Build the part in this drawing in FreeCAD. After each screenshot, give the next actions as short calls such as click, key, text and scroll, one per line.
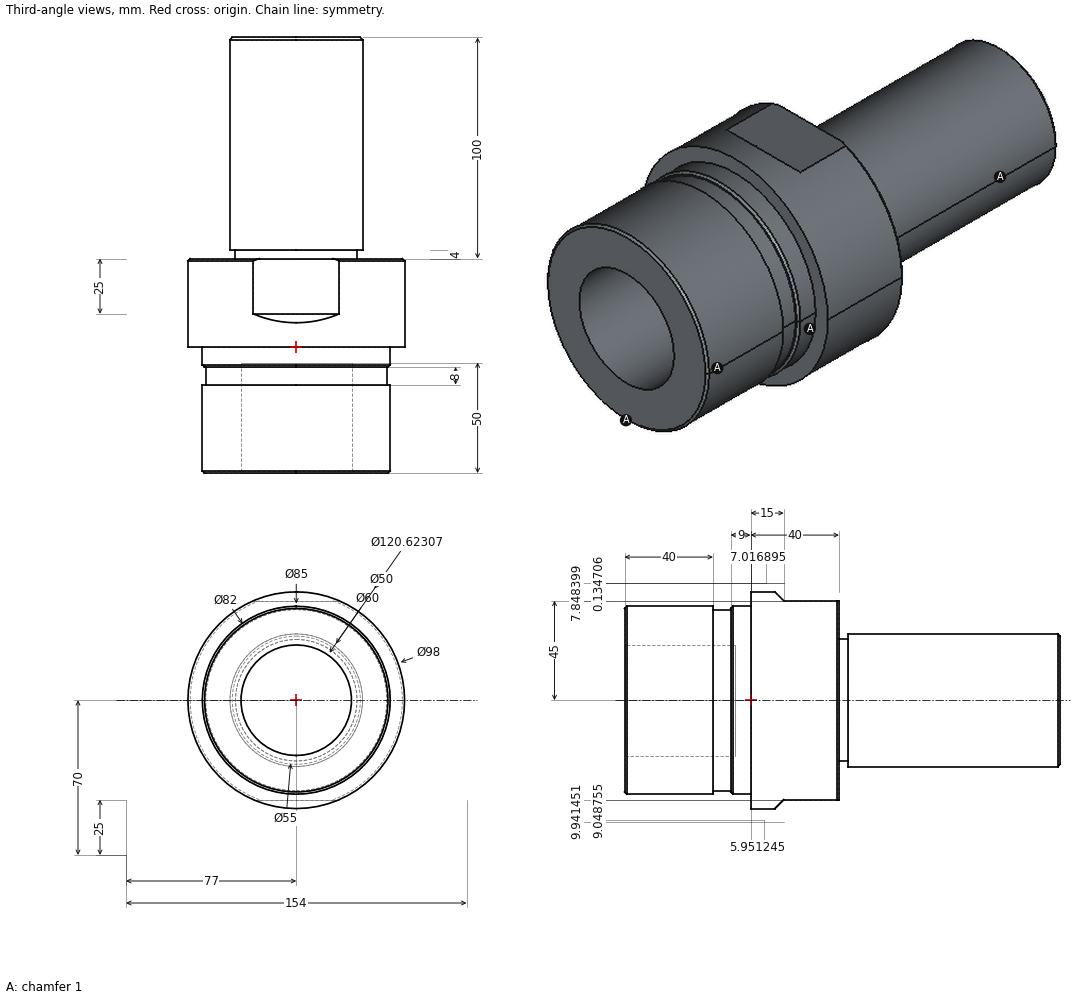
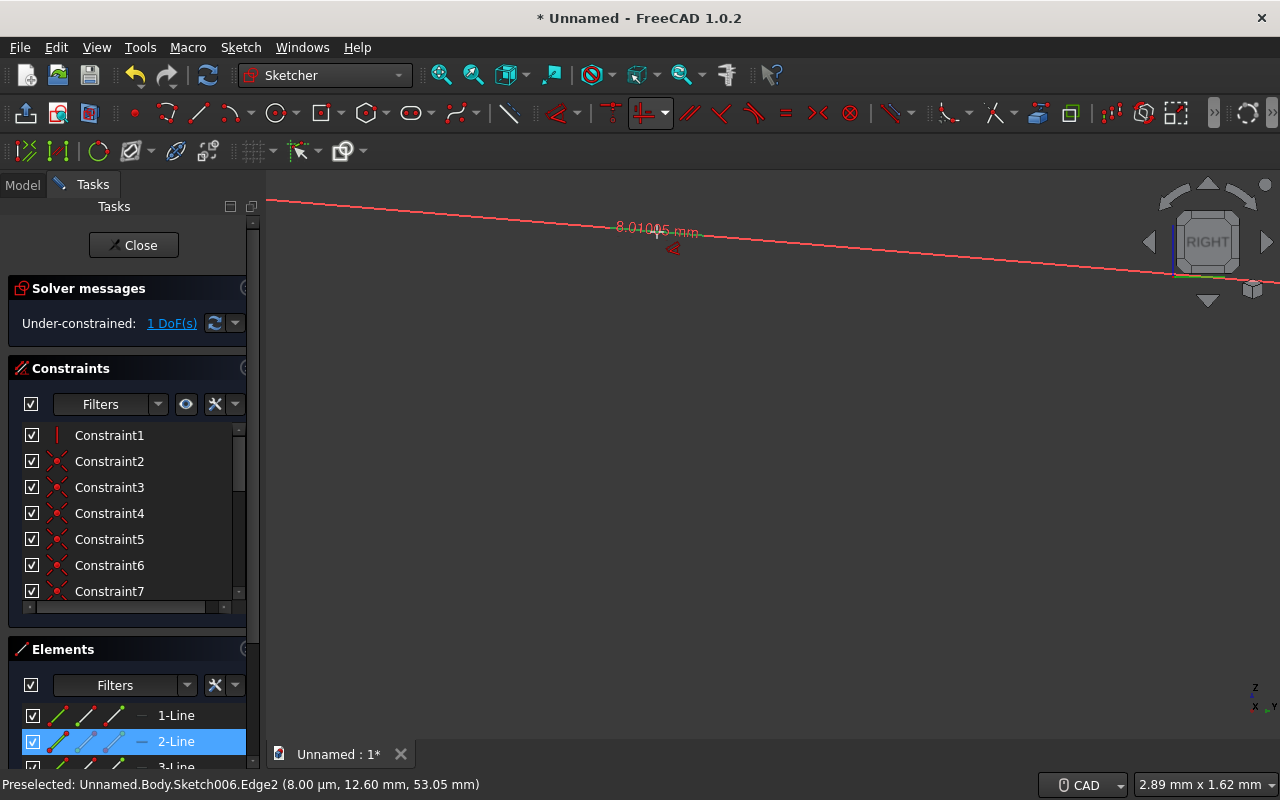
key(Escape)
key(Escape)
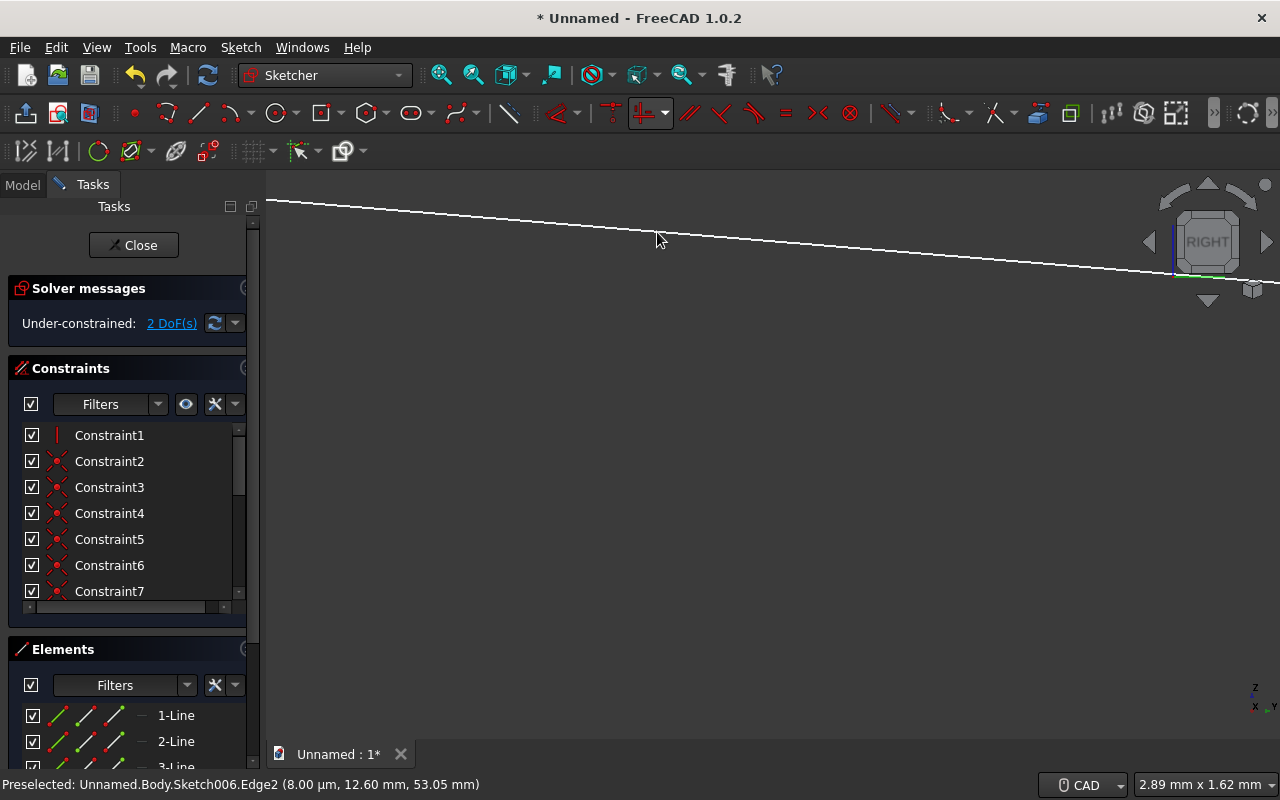
click(657, 232)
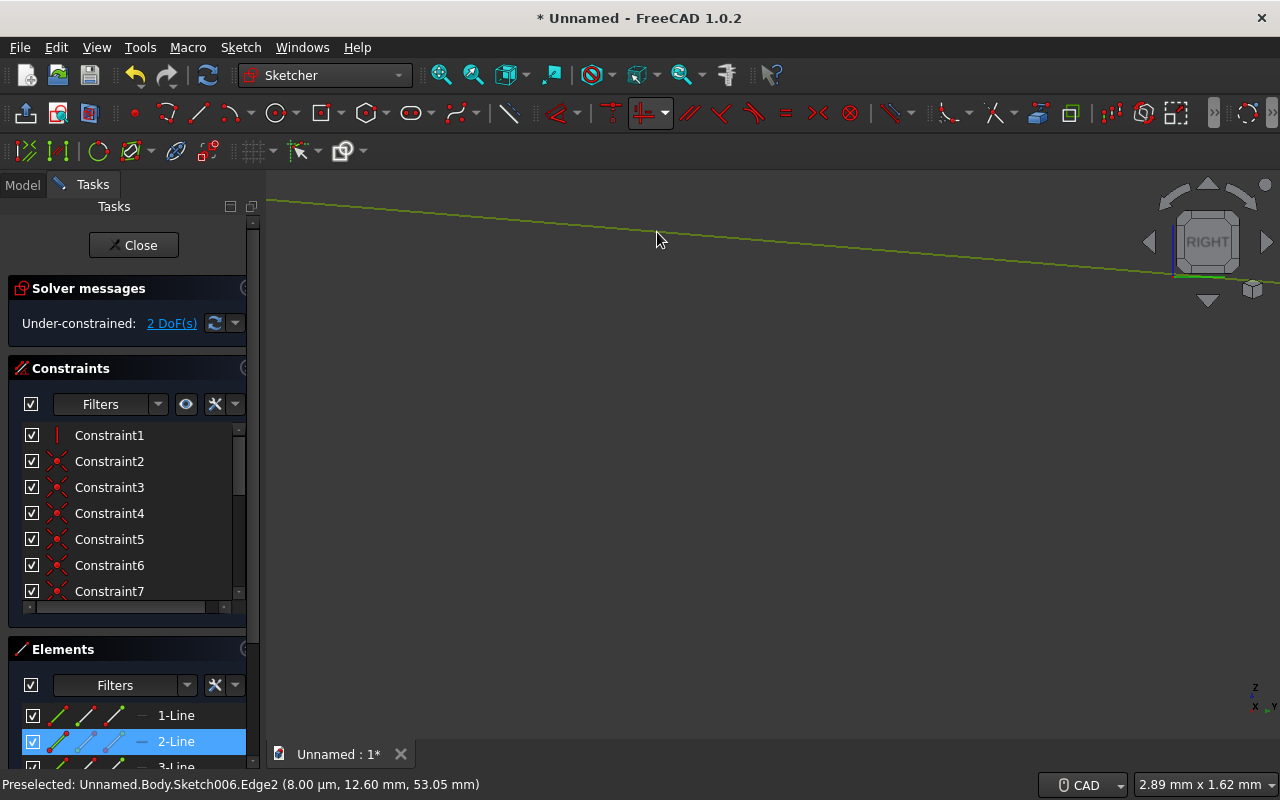
key(i)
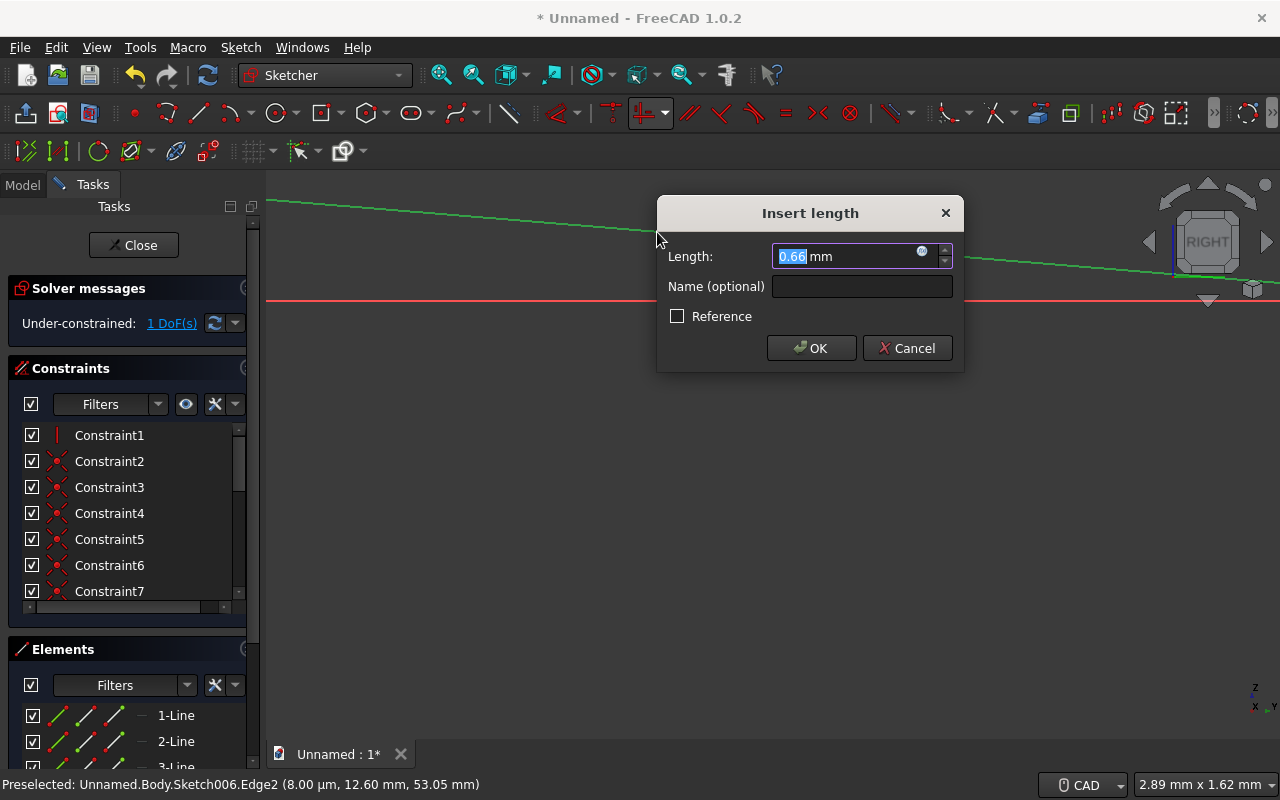
text(0.134706)
key(Return)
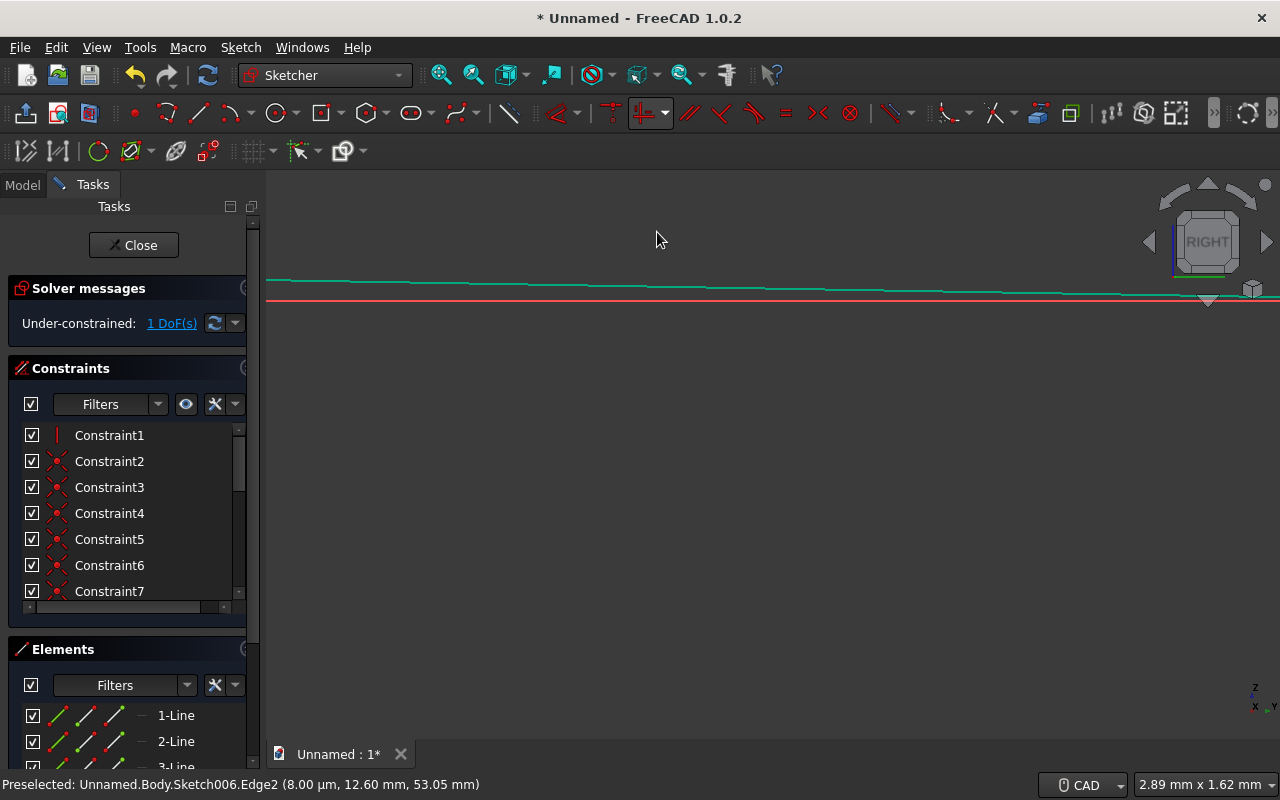
scroll(704, 454, down, 15)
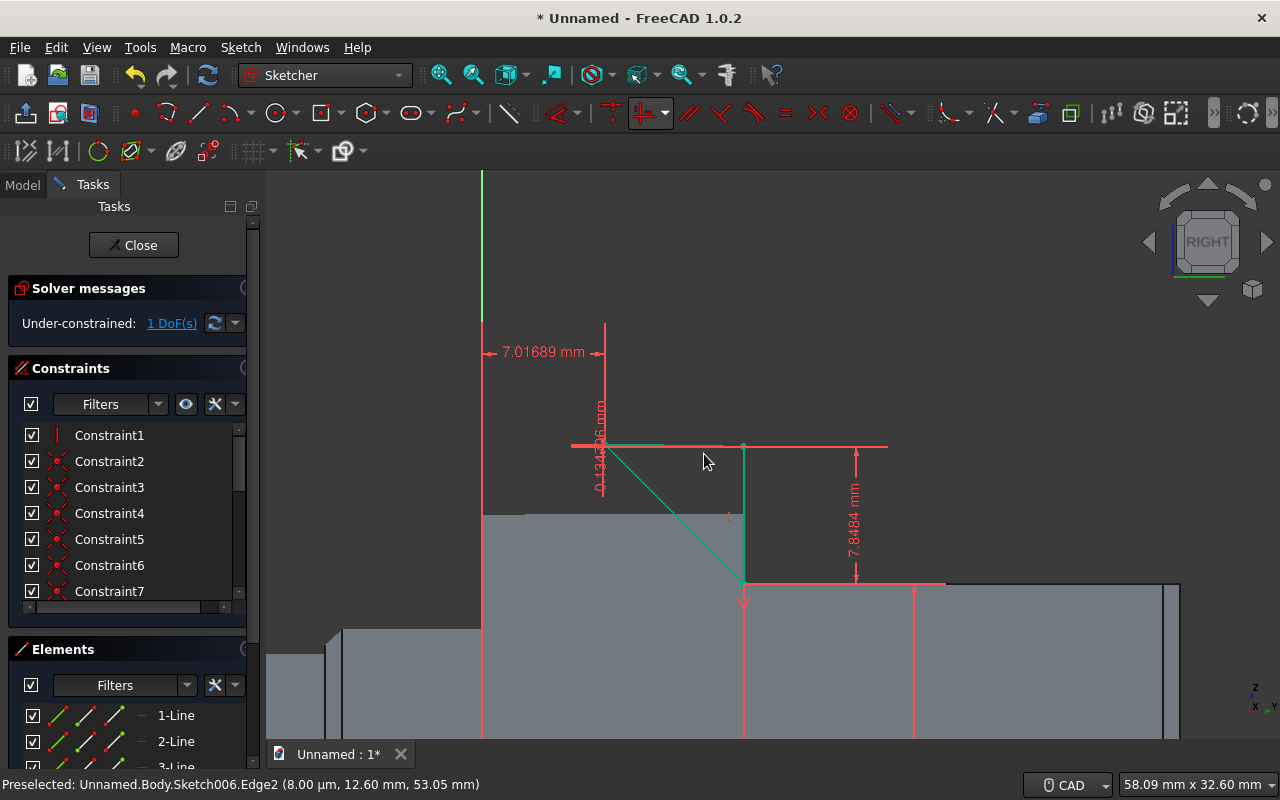
scroll(728, 219, down, 8)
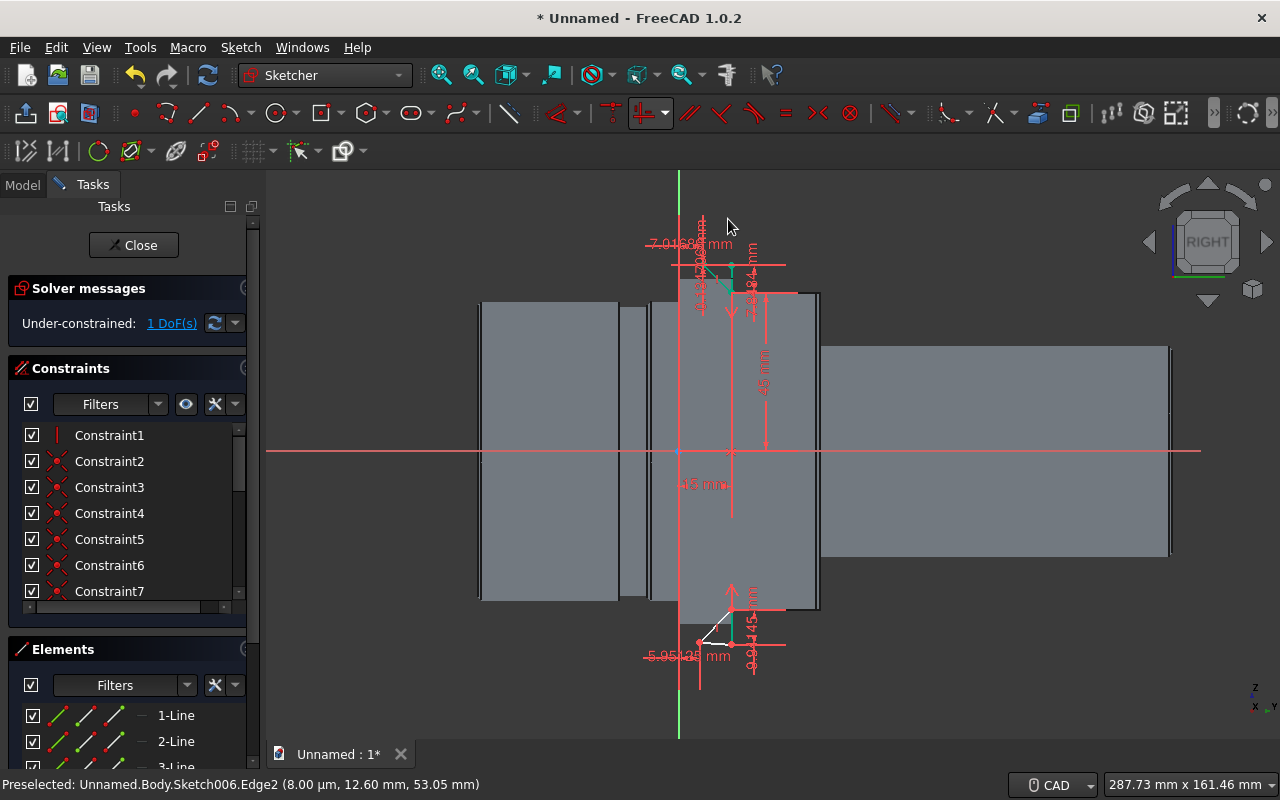
scroll(722, 620, up, 2)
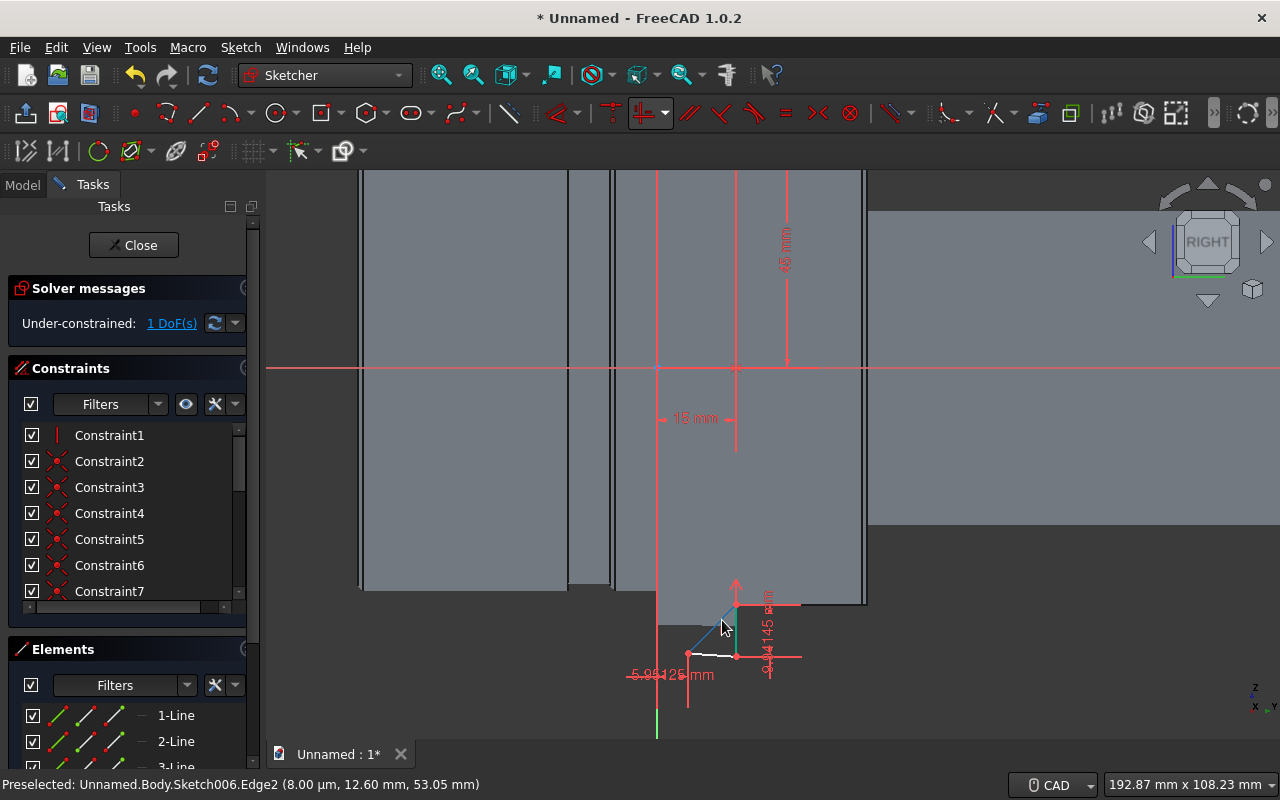
click(722, 619)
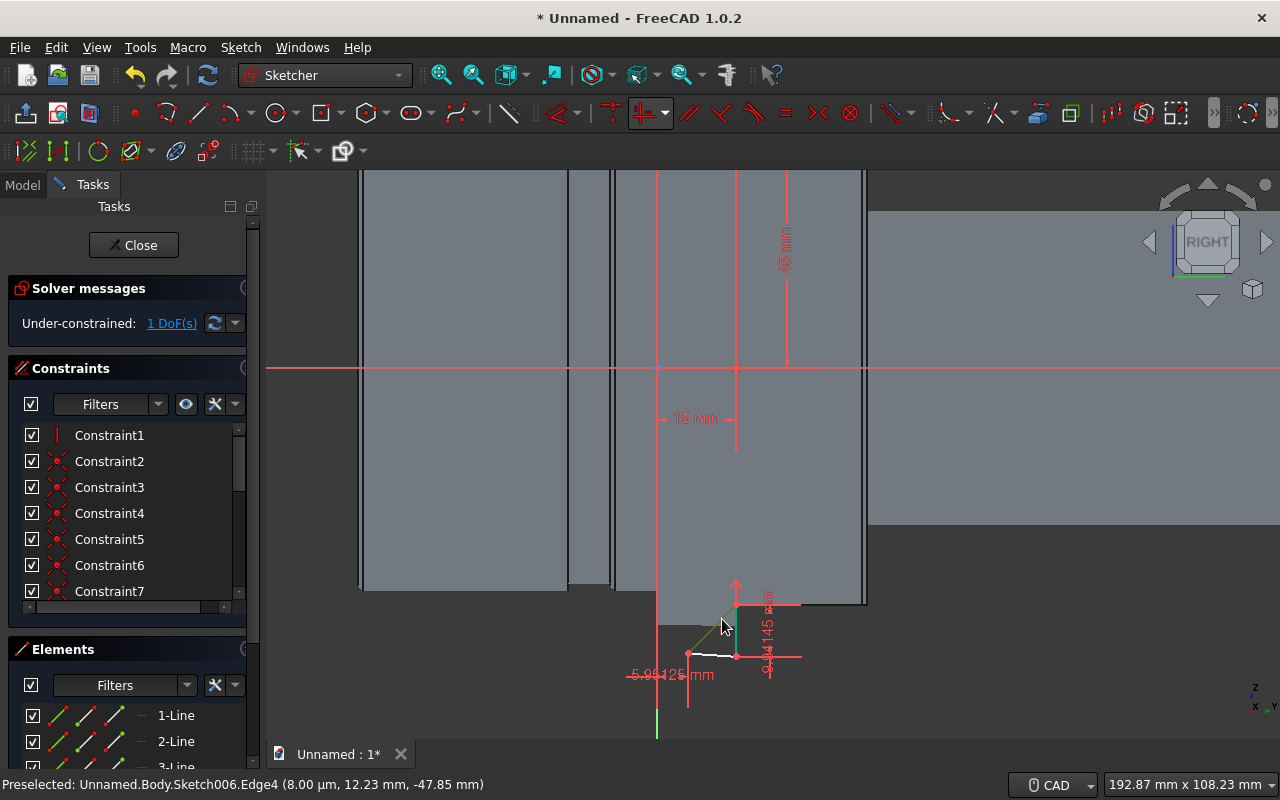
click(580, 114)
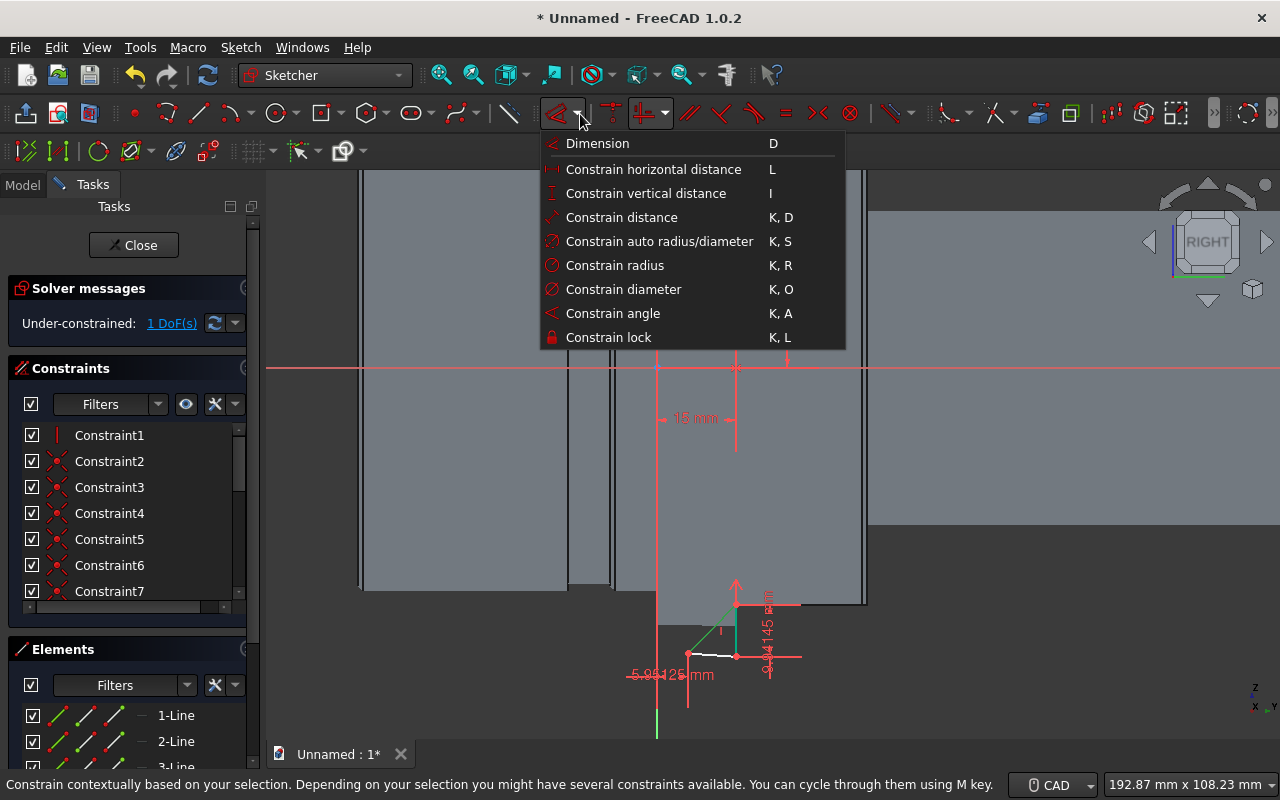
click(693, 193)